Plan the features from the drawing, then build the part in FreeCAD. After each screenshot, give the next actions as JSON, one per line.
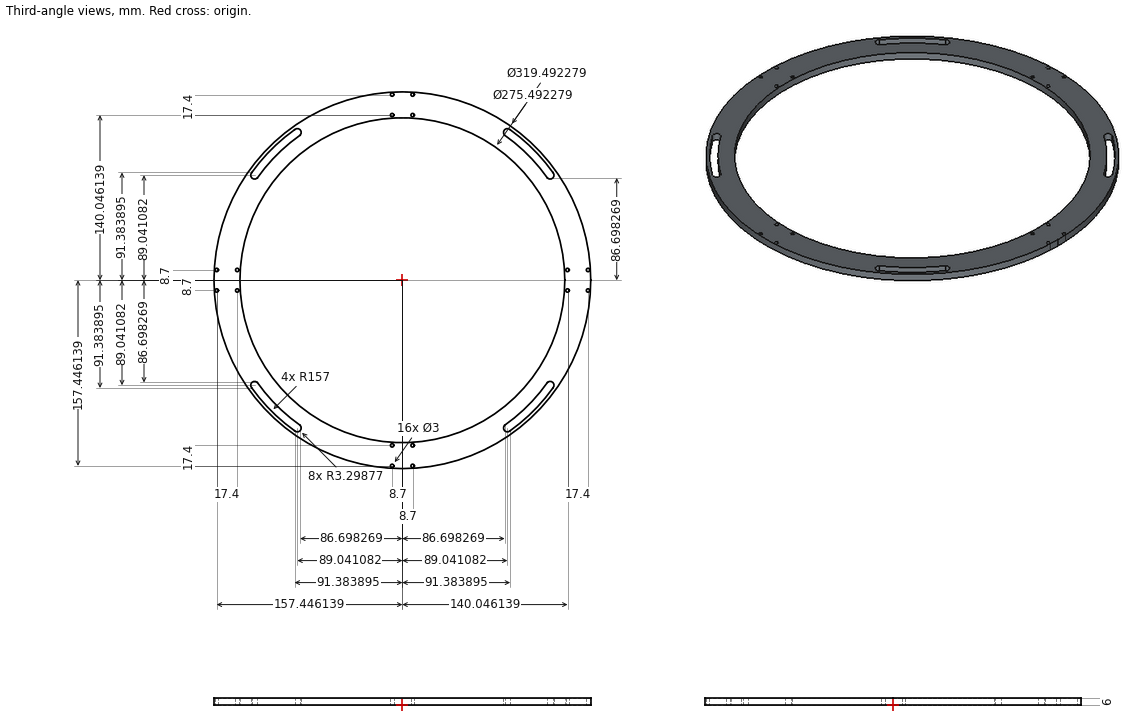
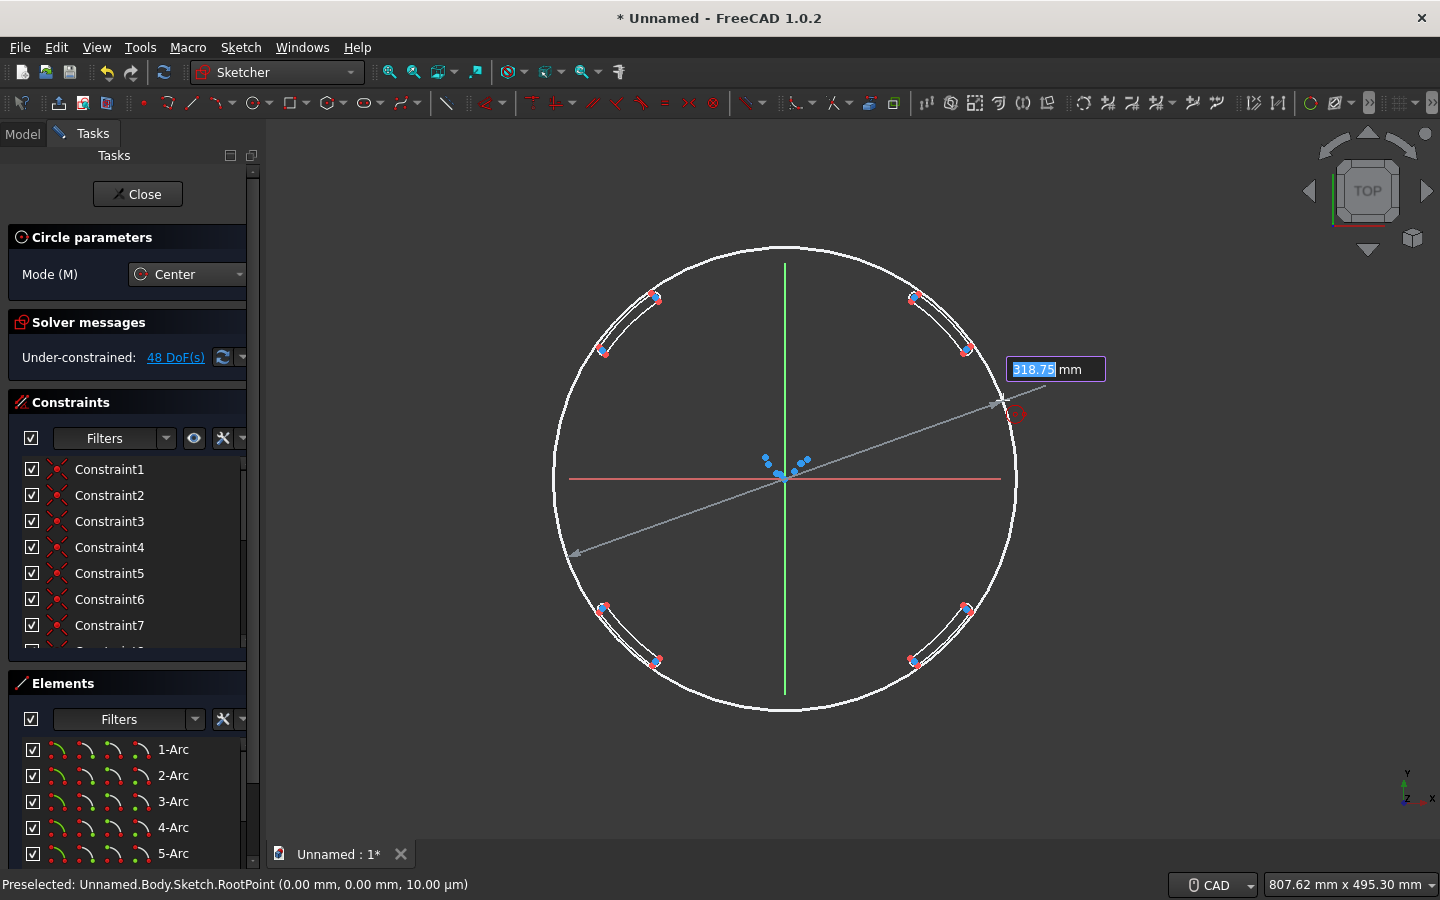
{"action": "type", "text": "319.492279"}
{"action": "key", "text": "Return"}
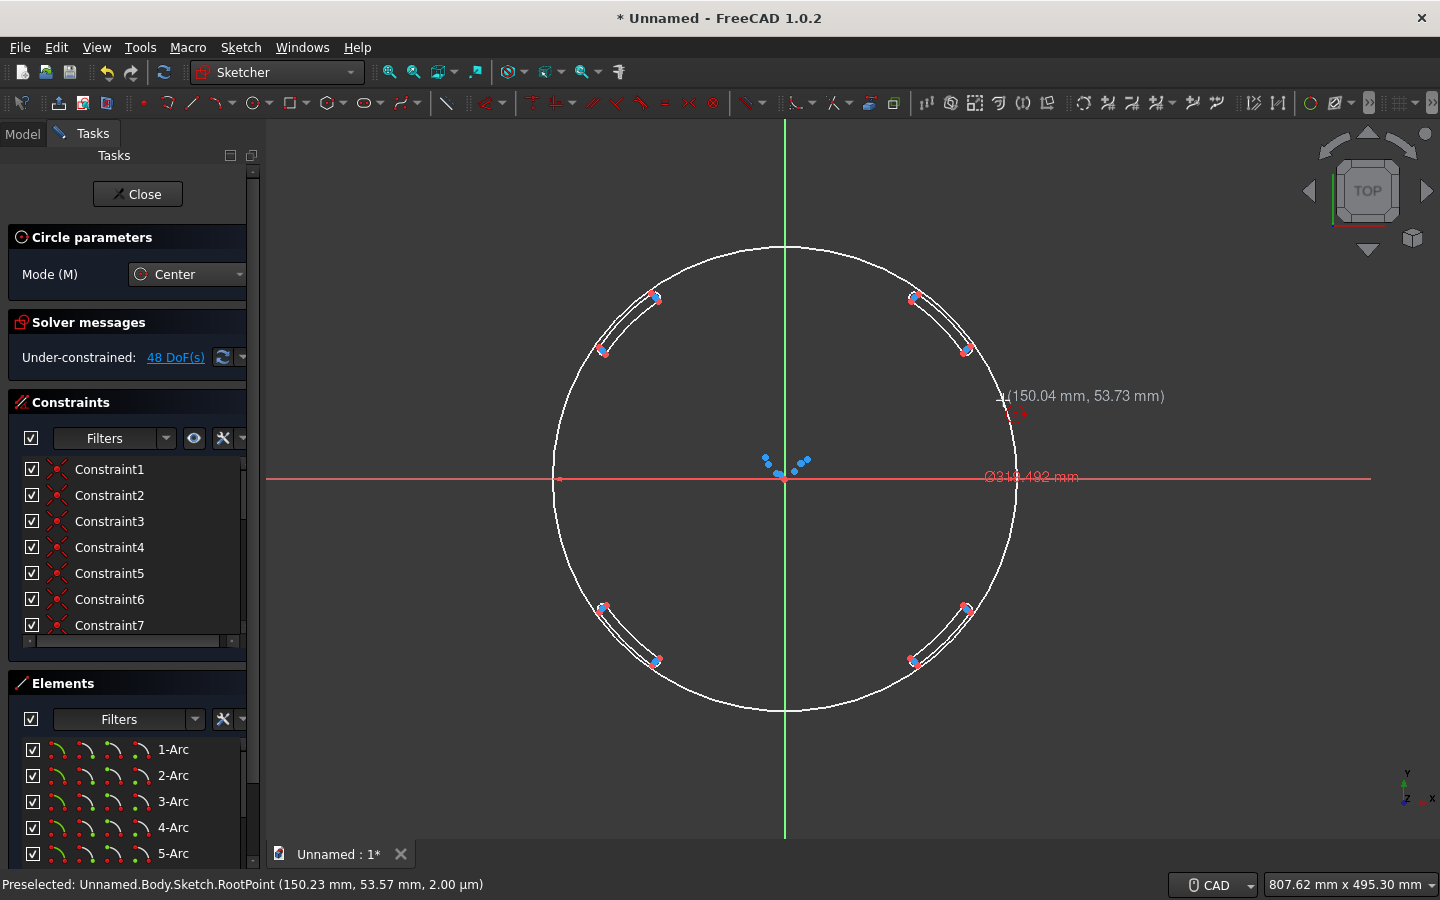
{"action": "scroll", "coordinate": [772, 708], "scroll_direction": "up", "scroll_amount": 12}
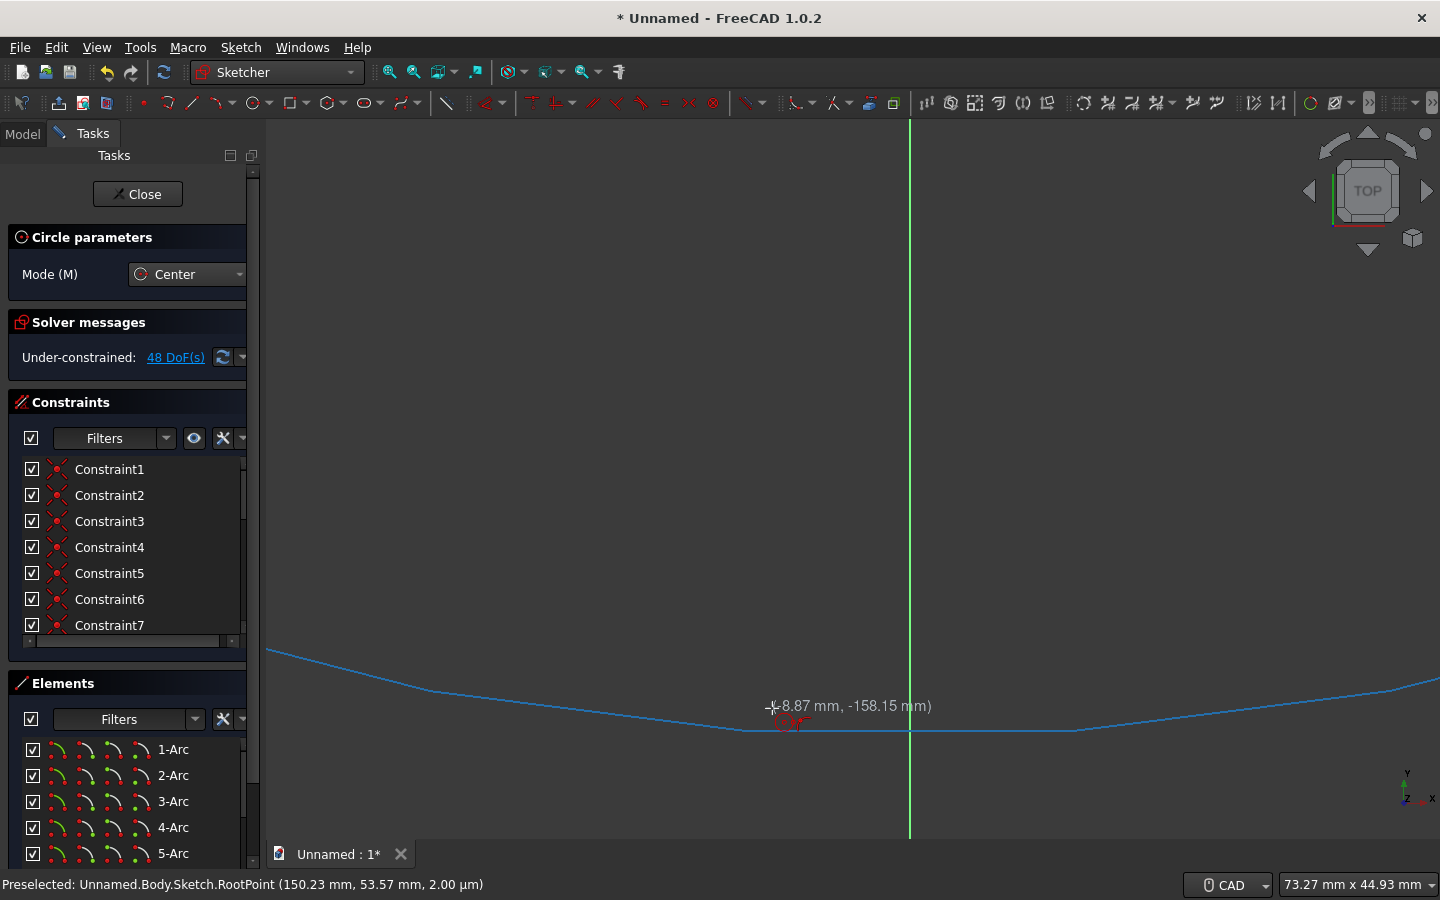
{"action": "left_click", "coordinate": [770, 700]}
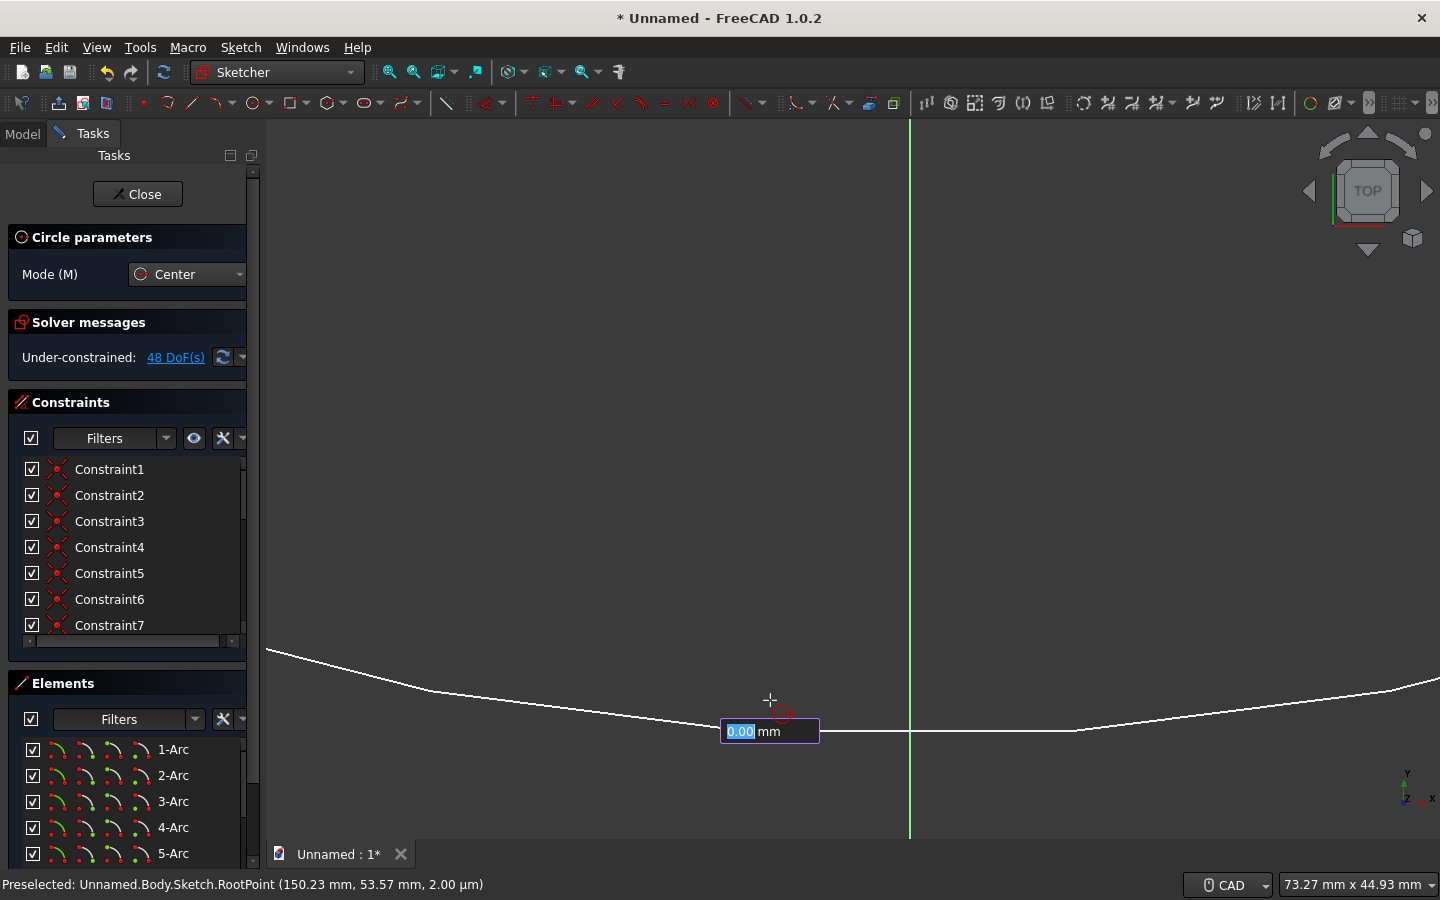
{"action": "scroll", "coordinate": [772, 709], "scroll_direction": "down", "scroll_amount": 12}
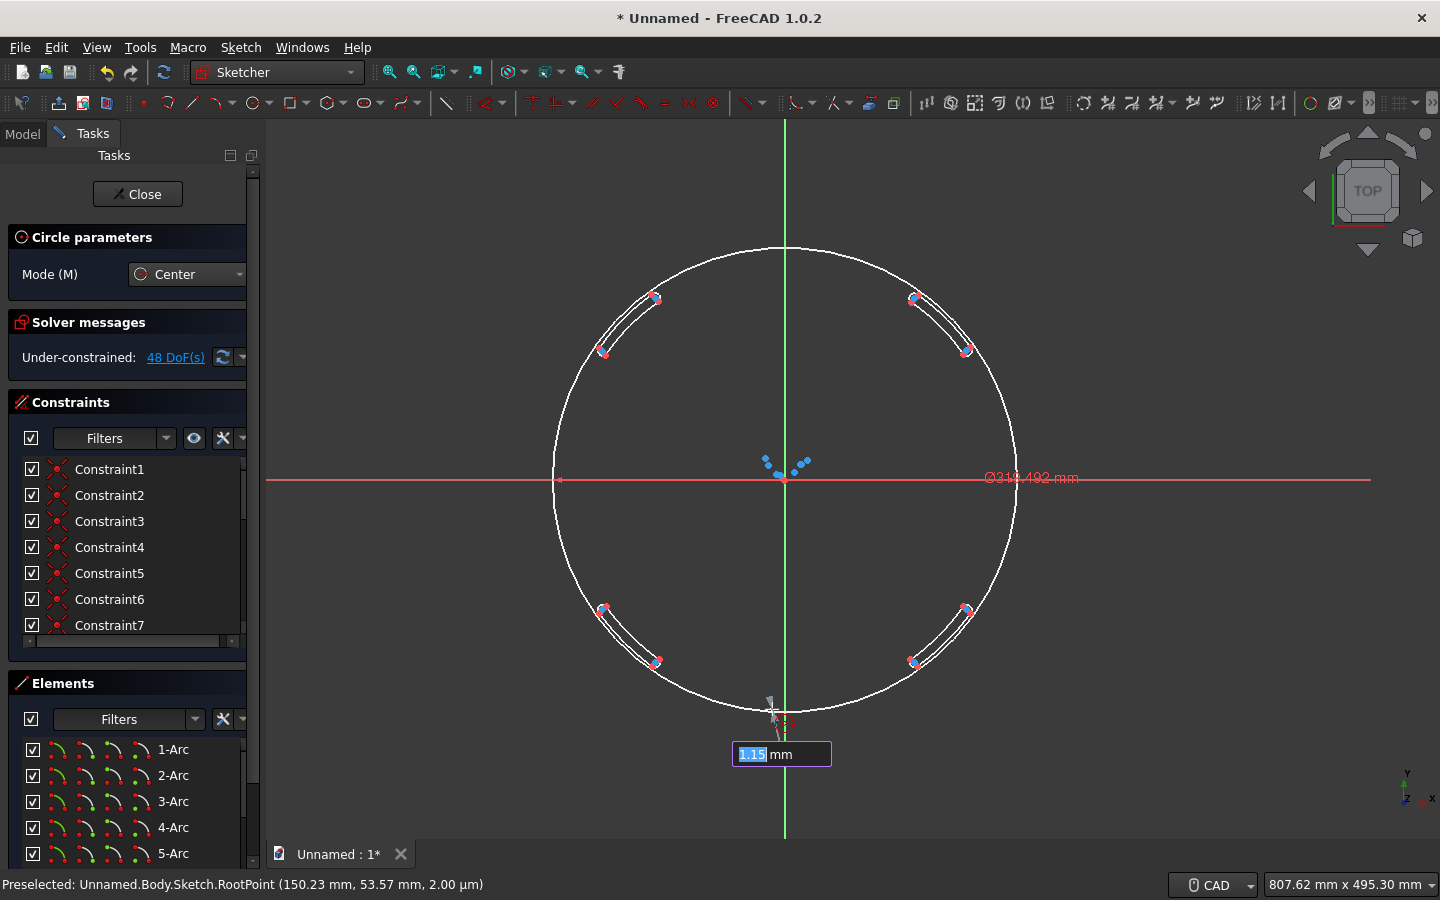
{"action": "scroll", "coordinate": [774, 707], "scroll_direction": "up", "scroll_amount": 7}
{"action": "mouse_move", "coordinate": [772, 706]}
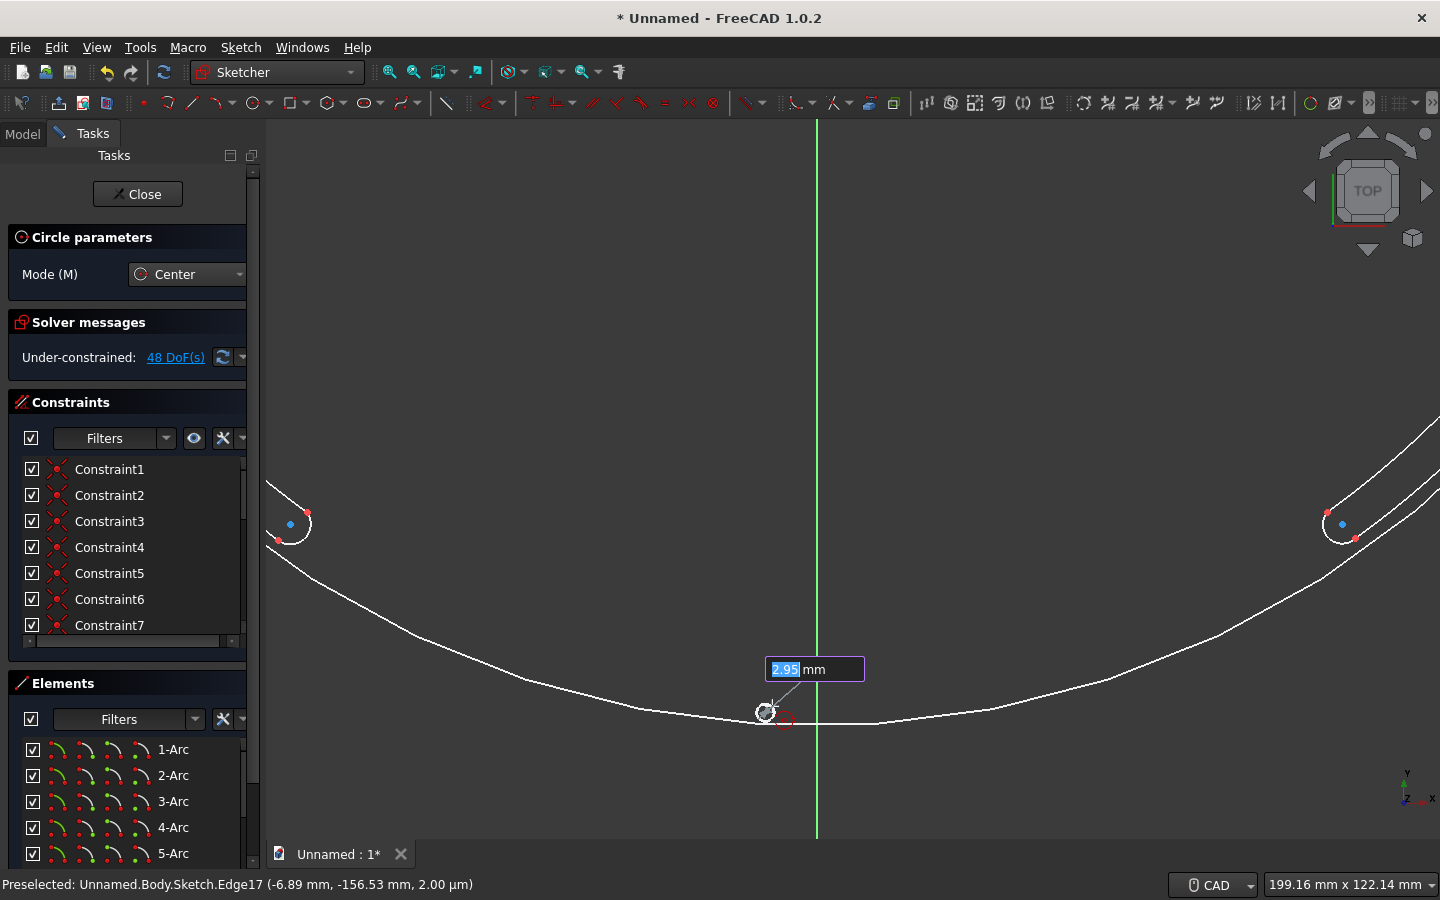
{"action": "type", "text": "3"}
{"action": "key", "text": "Return"}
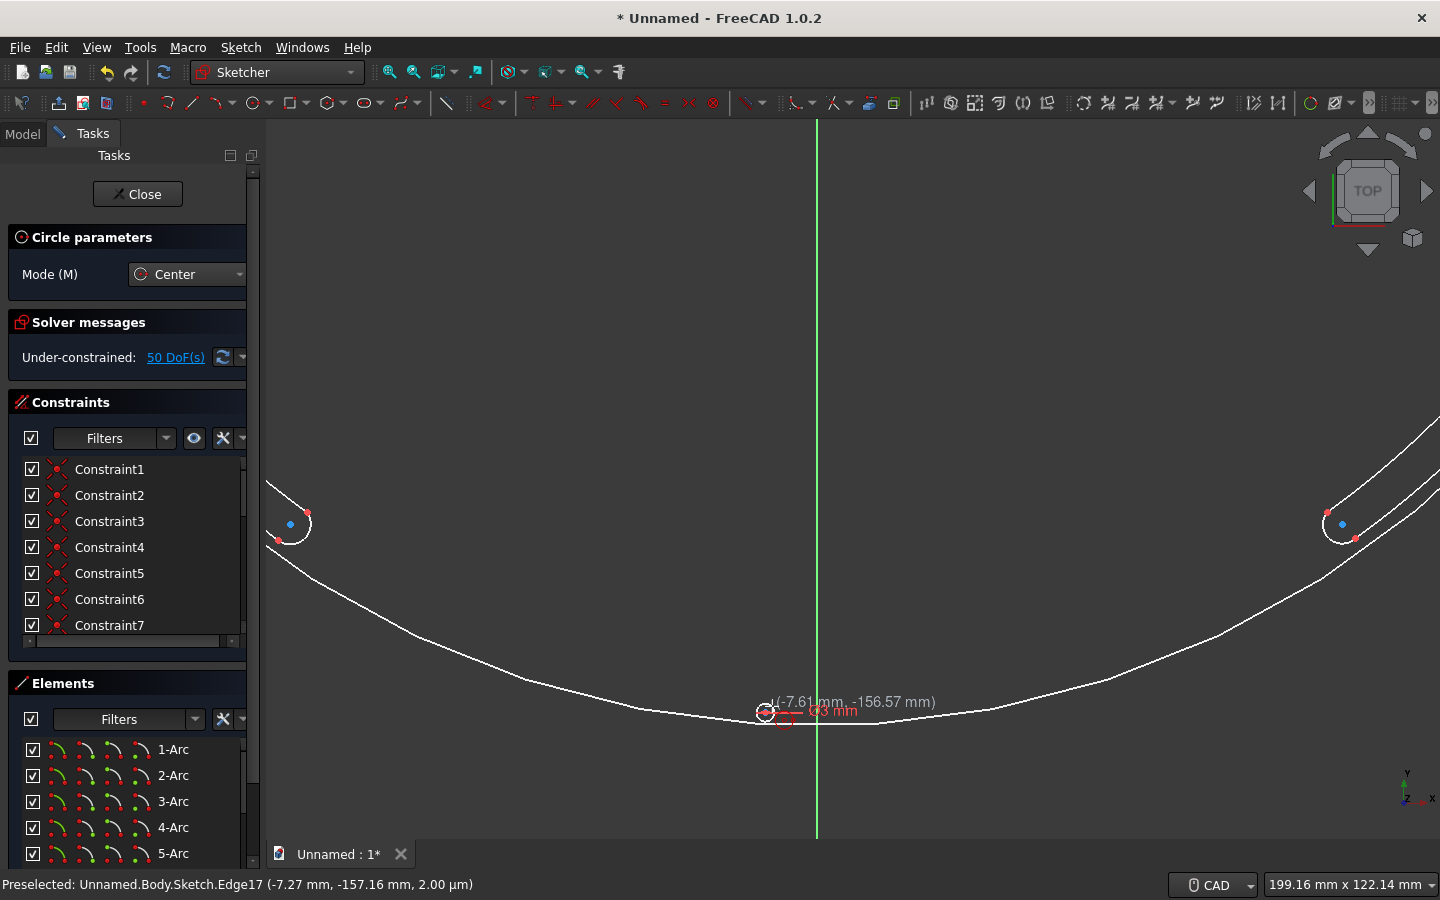
{"action": "scroll", "coordinate": [766, 610], "scroll_direction": "up", "scroll_amount": 5}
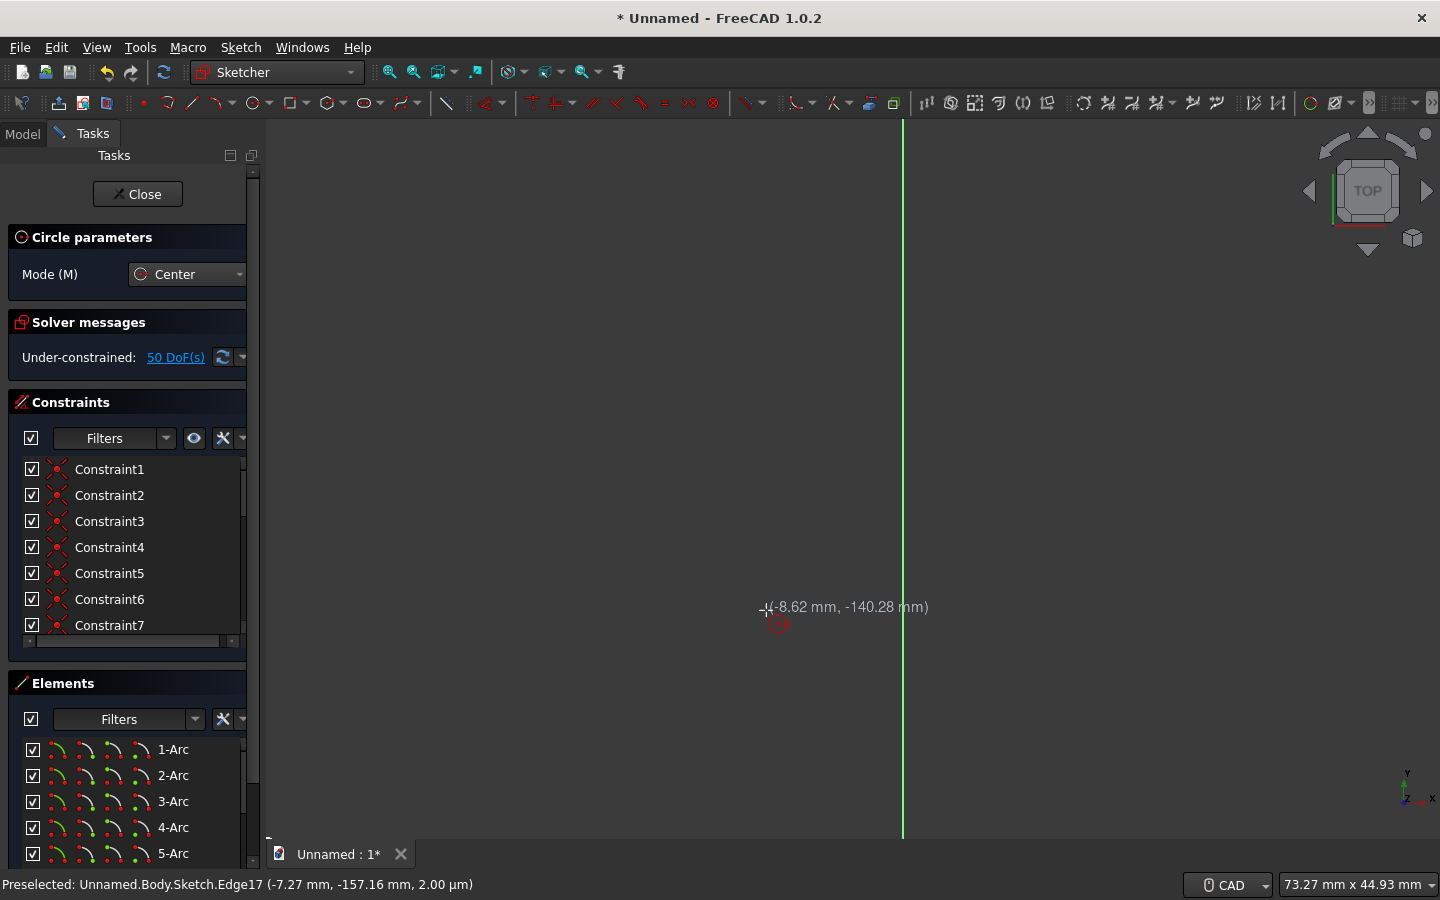
{"action": "scroll", "coordinate": [773, 690], "scroll_direction": "down", "scroll_amount": 12}